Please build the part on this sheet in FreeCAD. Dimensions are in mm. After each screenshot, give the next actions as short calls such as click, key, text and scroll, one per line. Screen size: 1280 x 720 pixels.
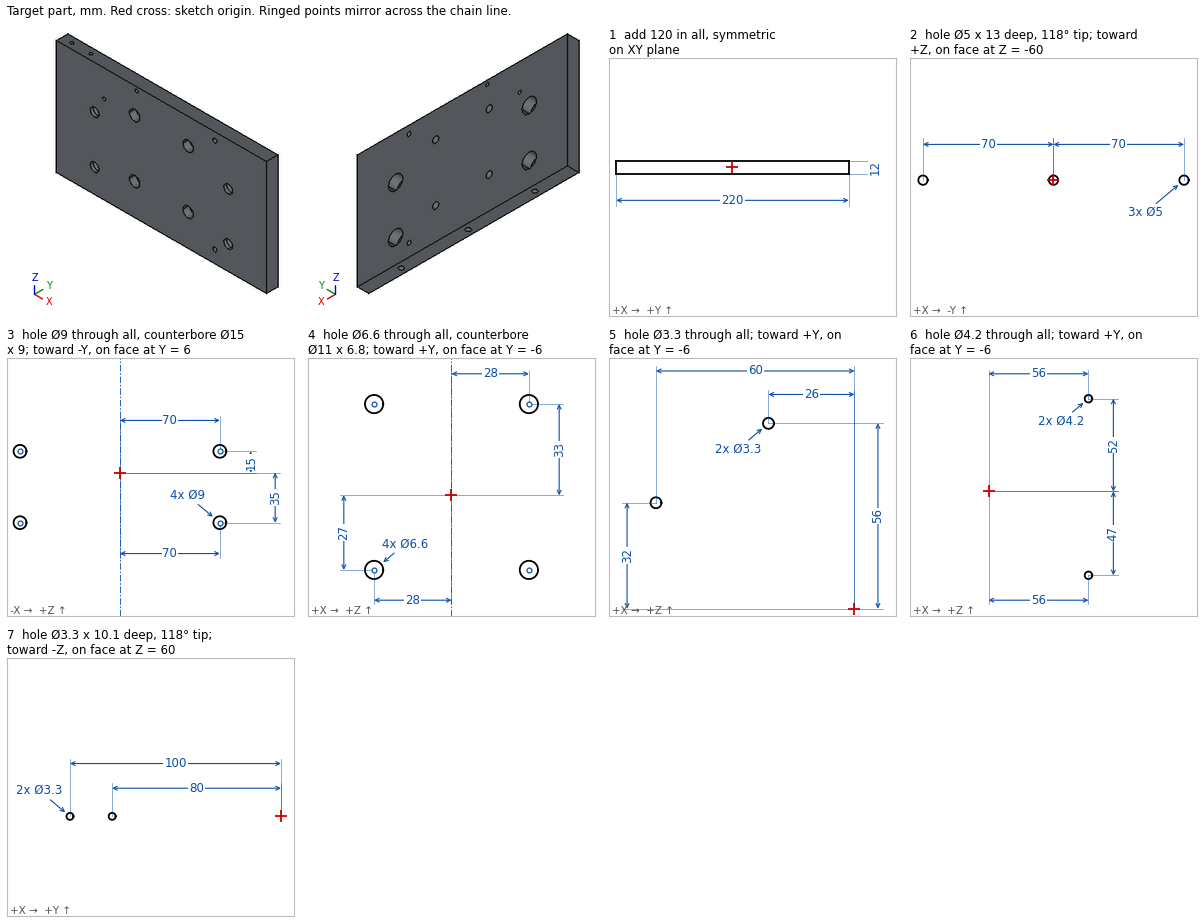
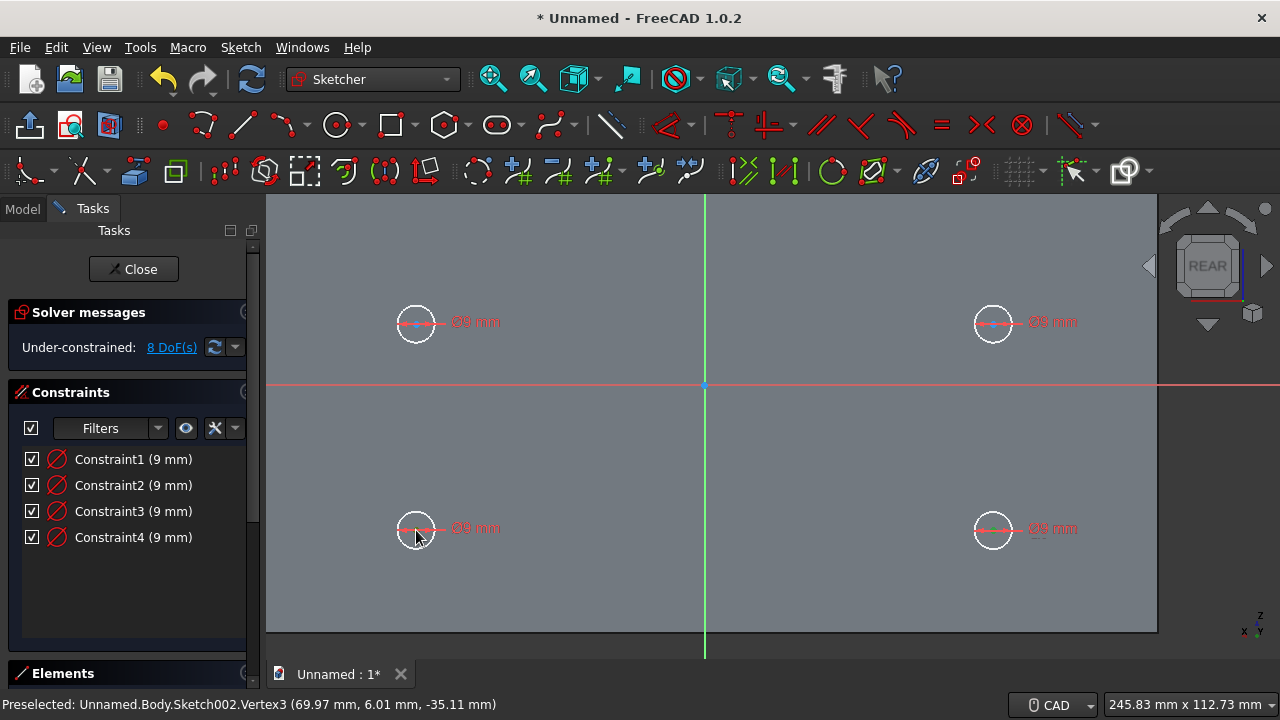
click(705, 602)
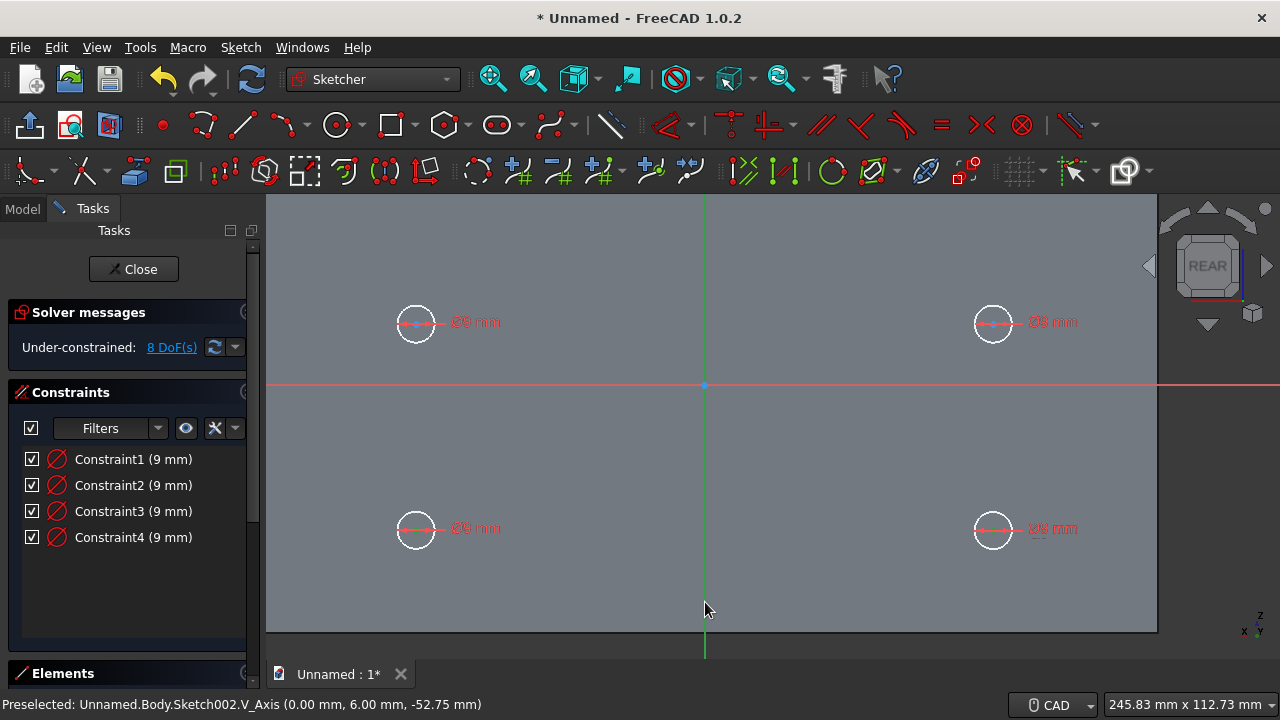
click(982, 126)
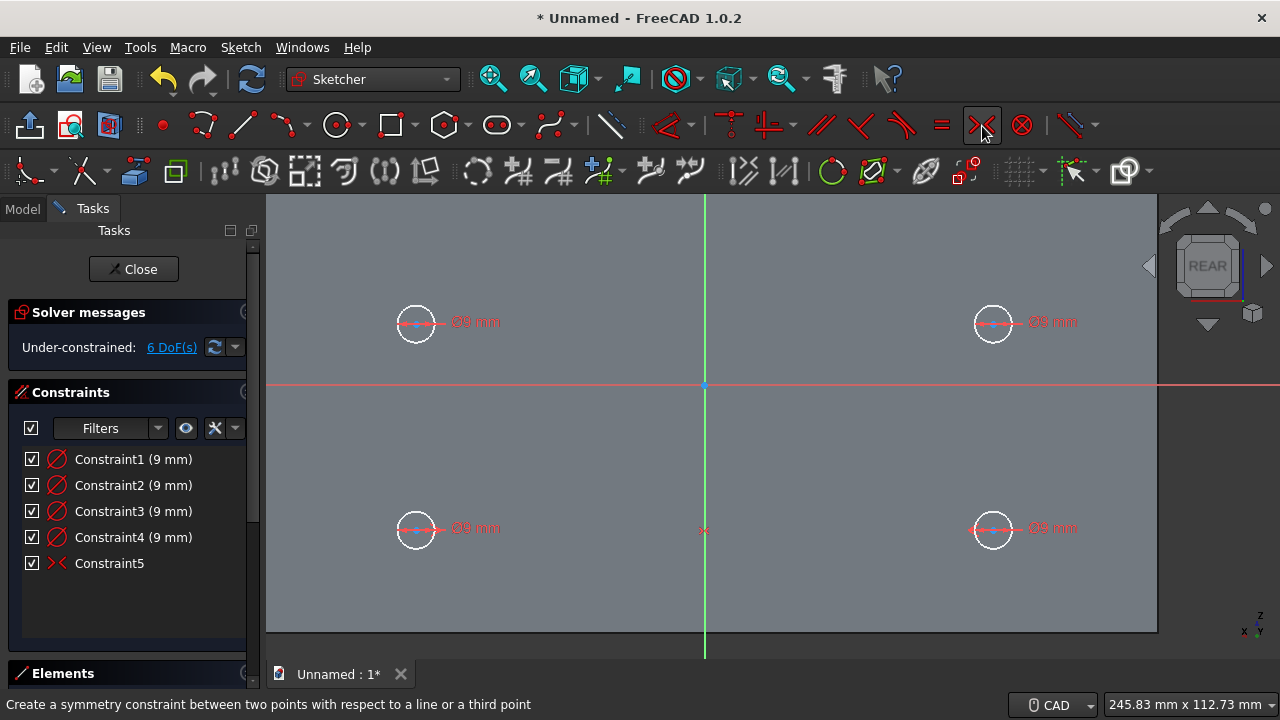
click(993, 324)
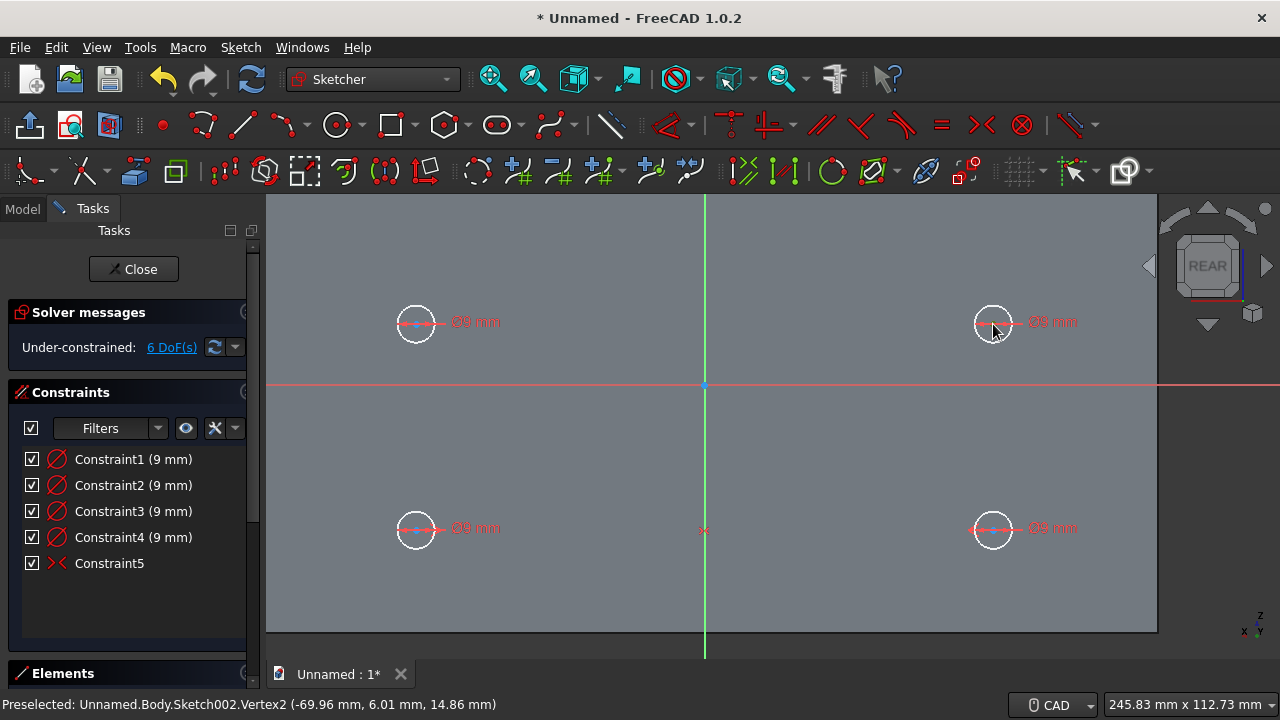
click(416, 324)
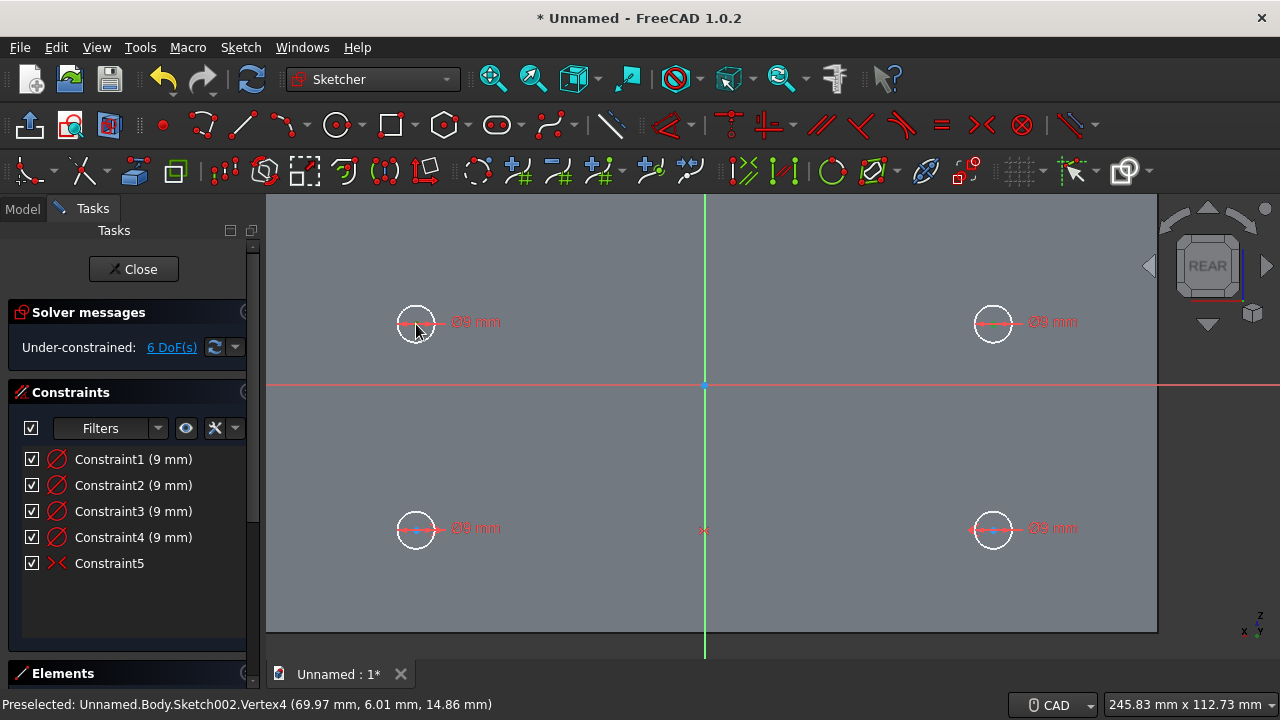
click(705, 602)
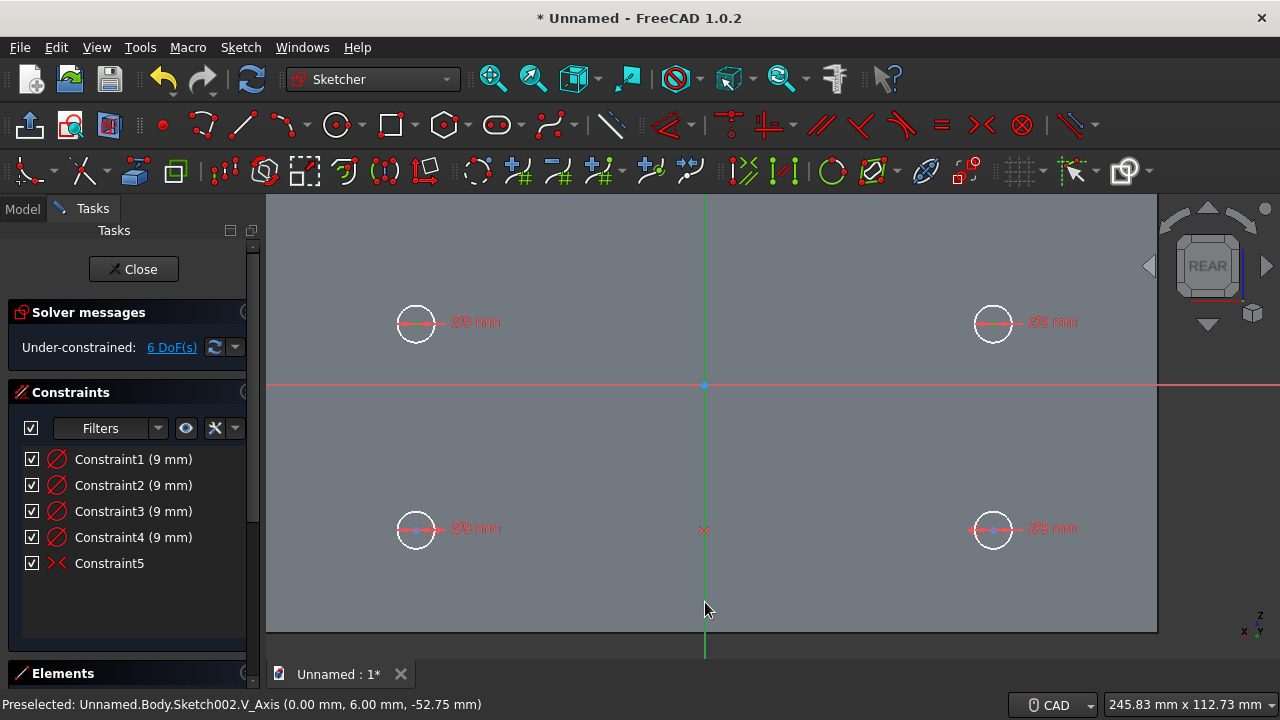
key(s)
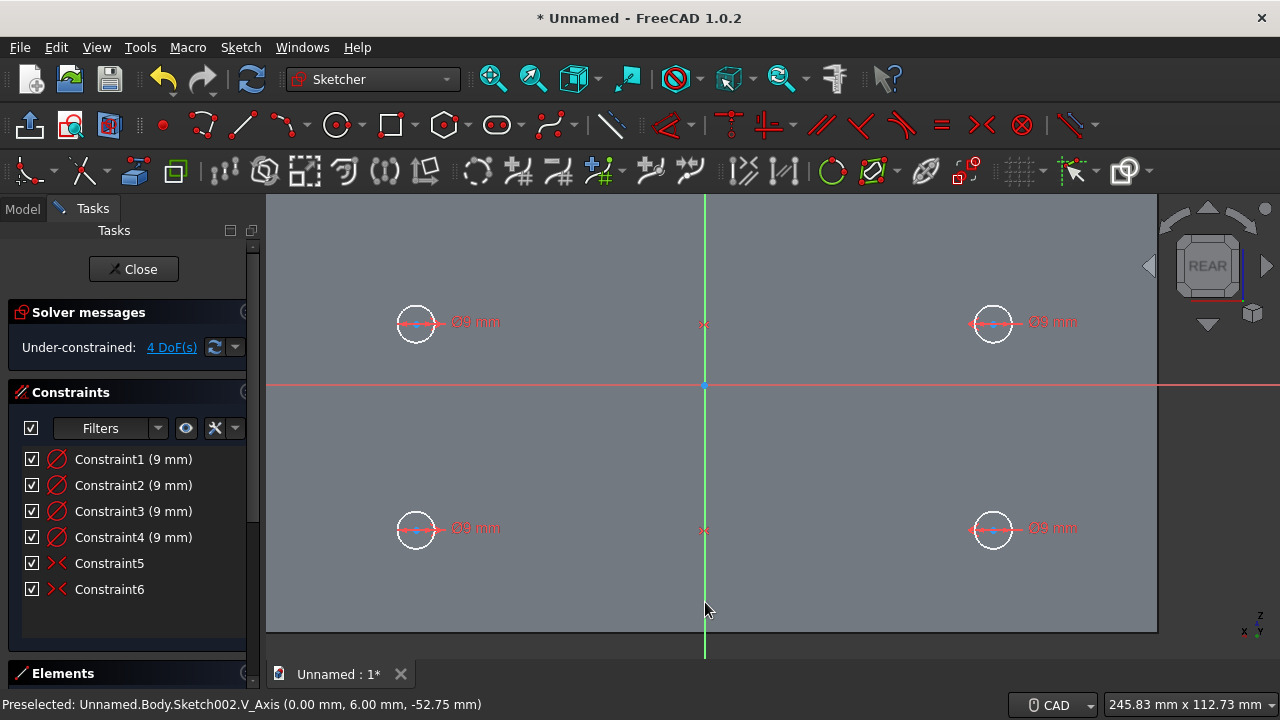
click(666, 126)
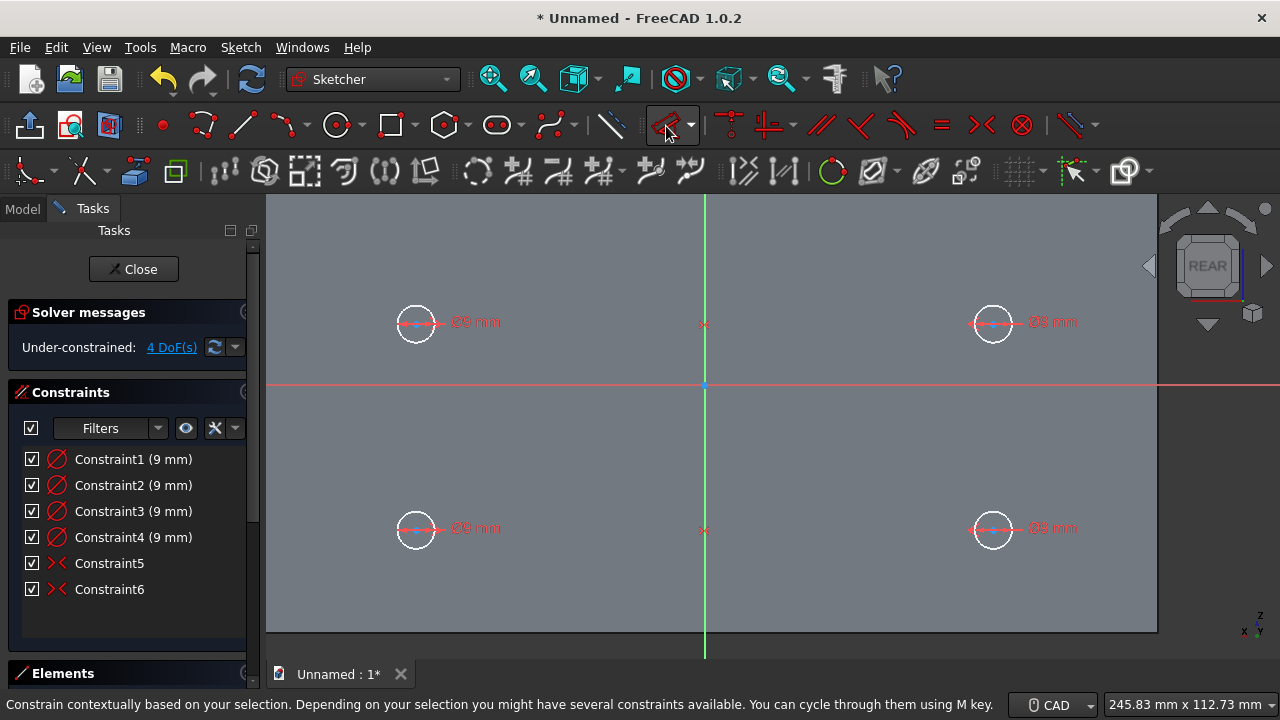
click(993, 530)
click(849, 564)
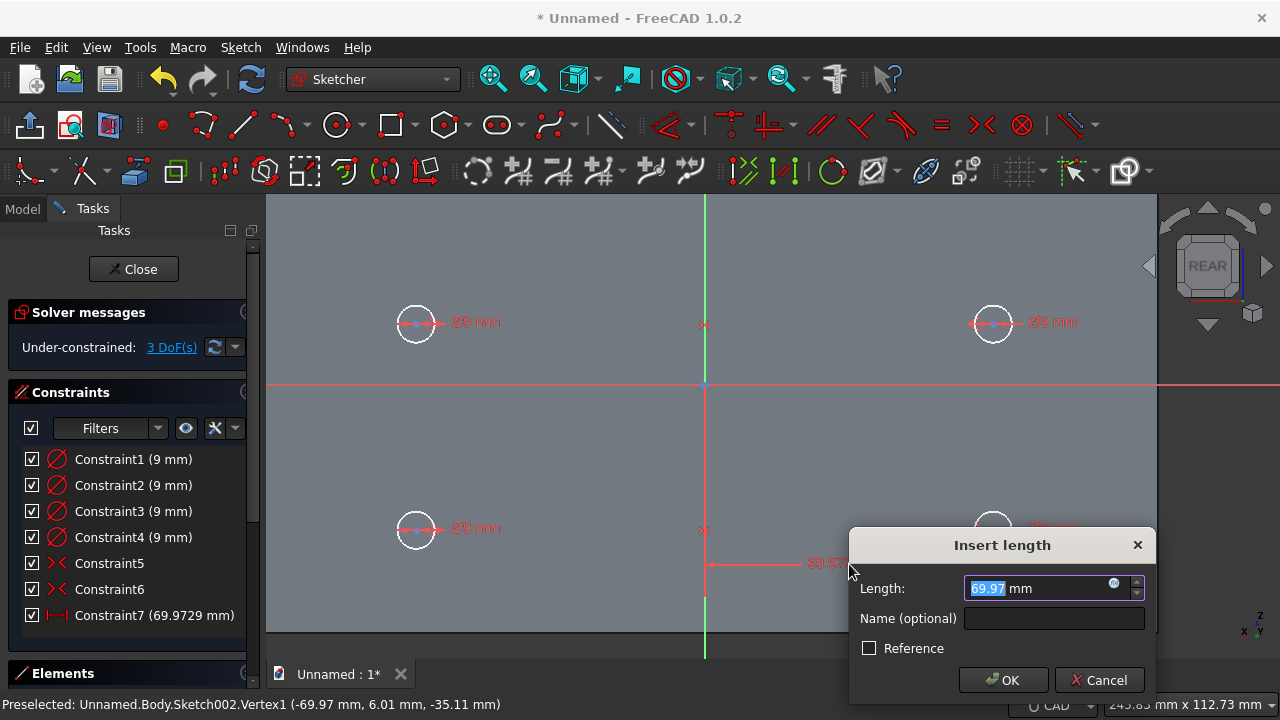
text(70)
key(Return)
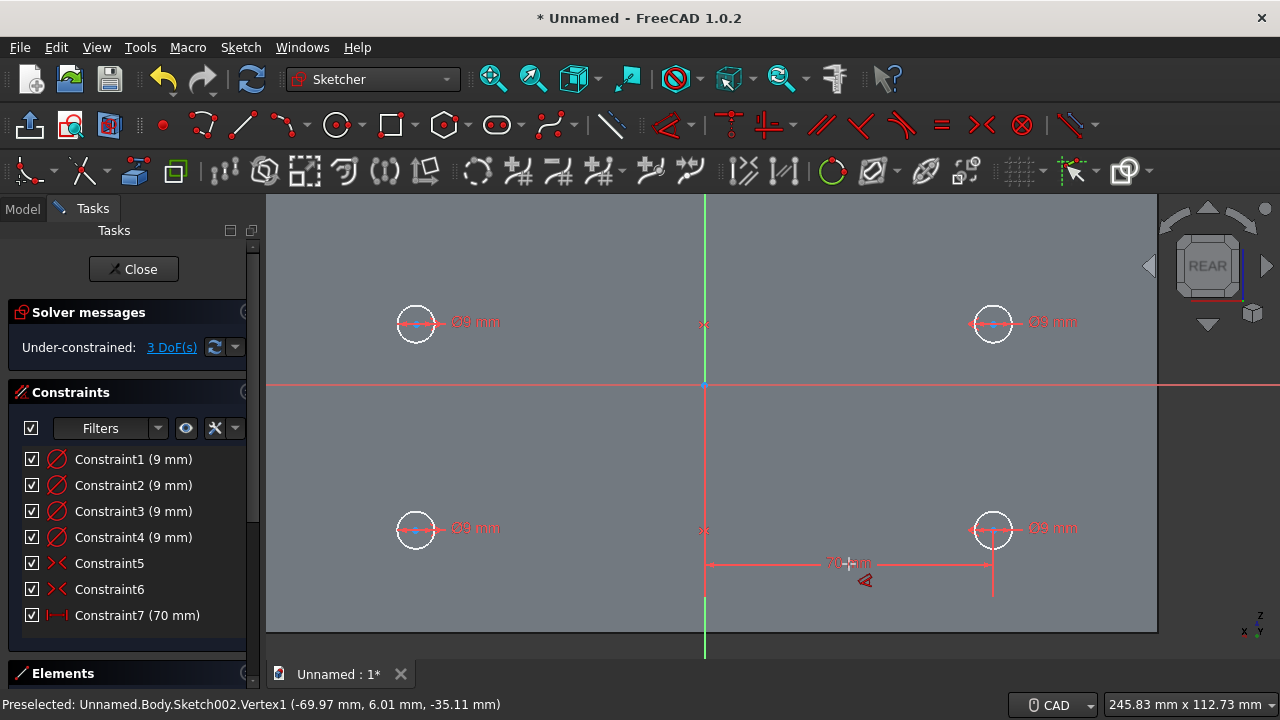
click(993, 530)
click(1027, 458)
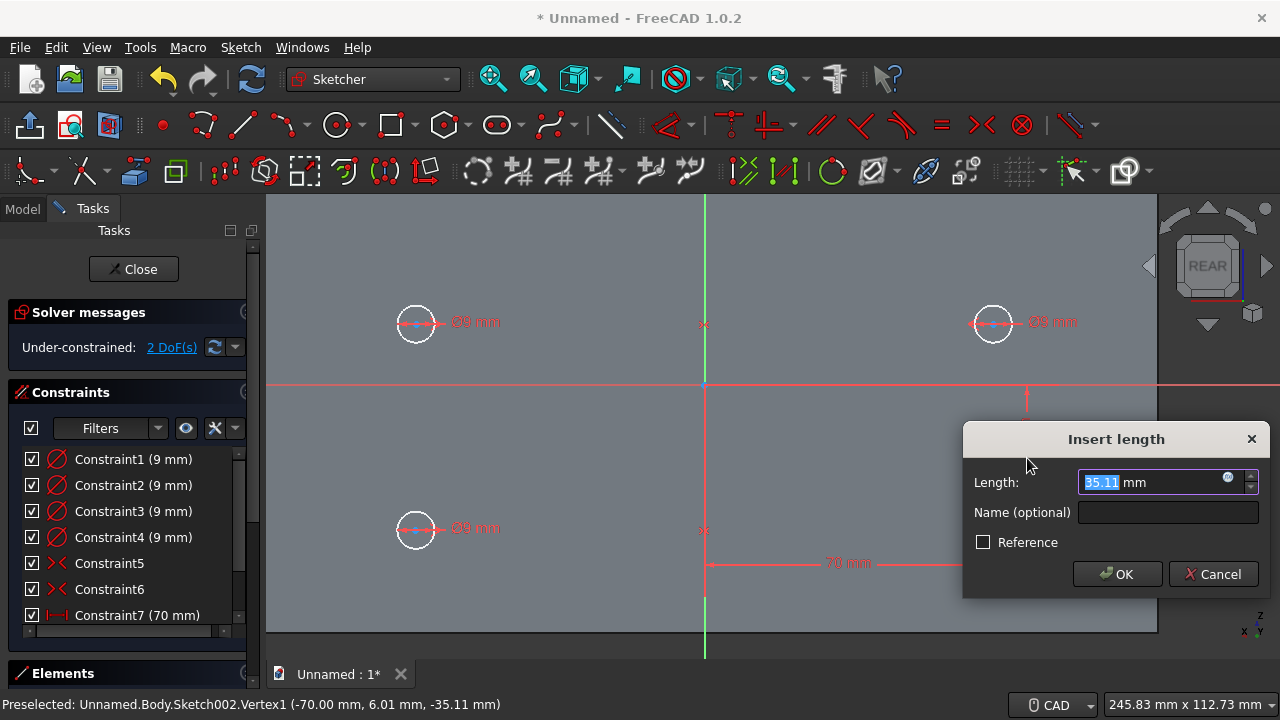
text(35)
key(Return)